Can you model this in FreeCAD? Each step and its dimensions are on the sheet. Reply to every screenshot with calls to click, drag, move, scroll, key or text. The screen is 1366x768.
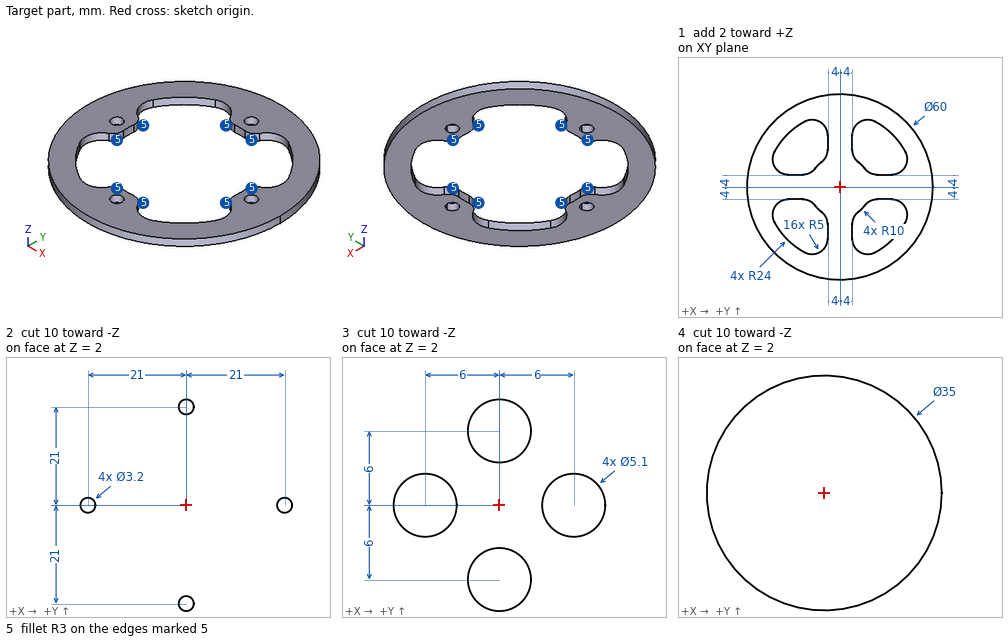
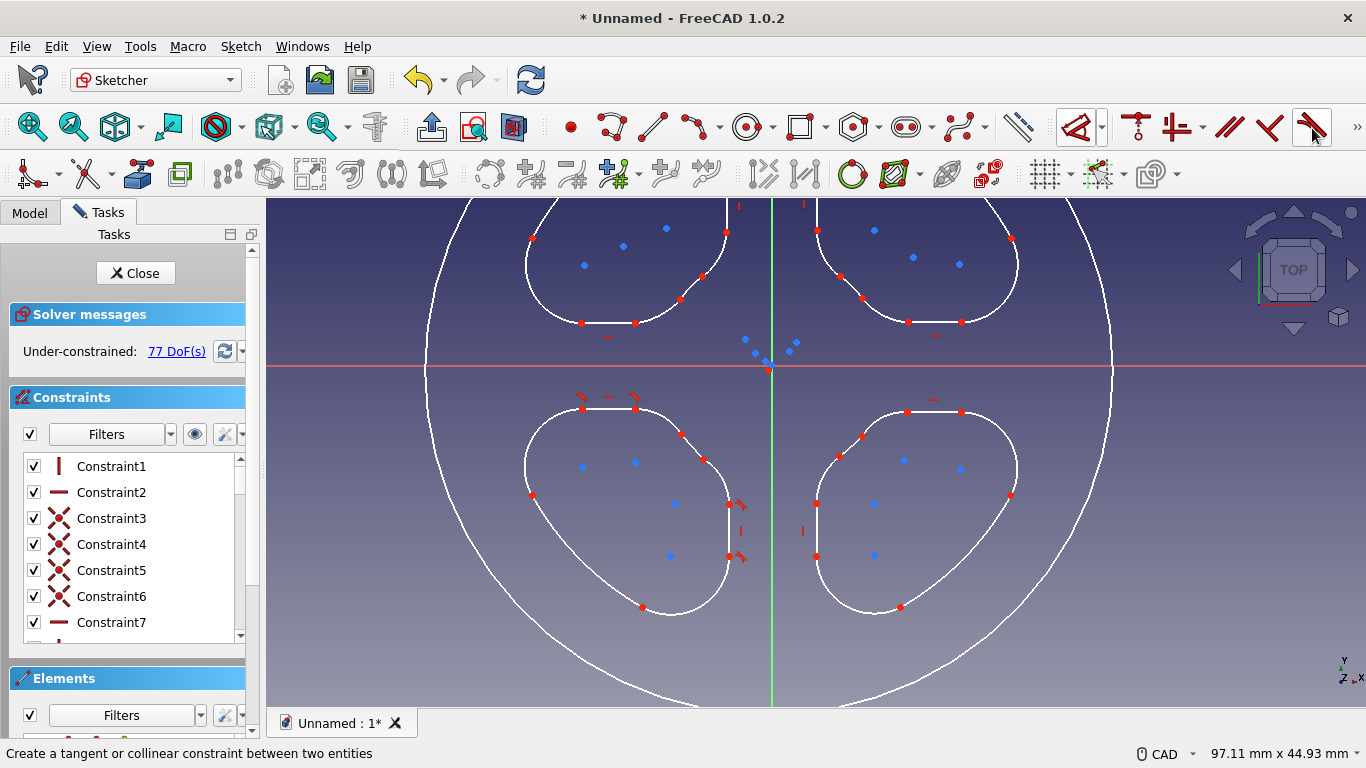
click(678, 614)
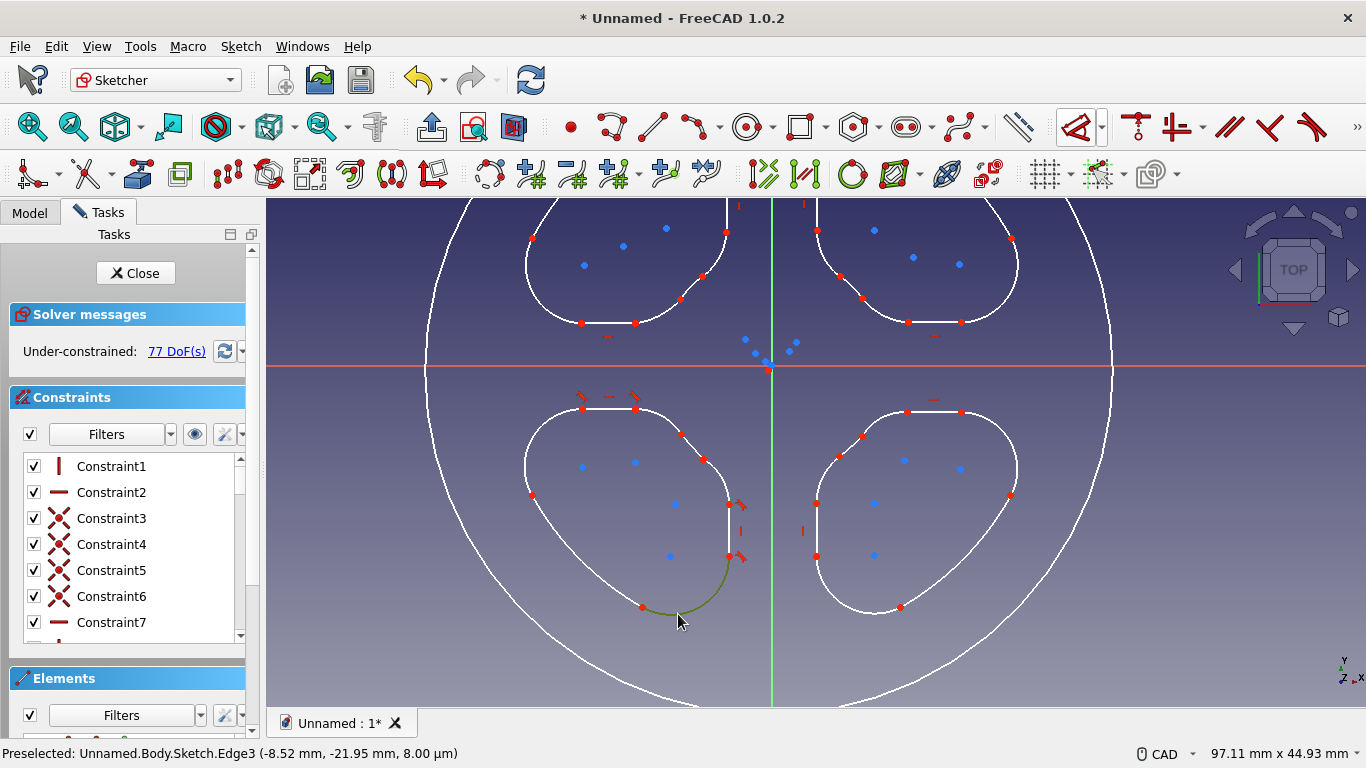
click(559, 535)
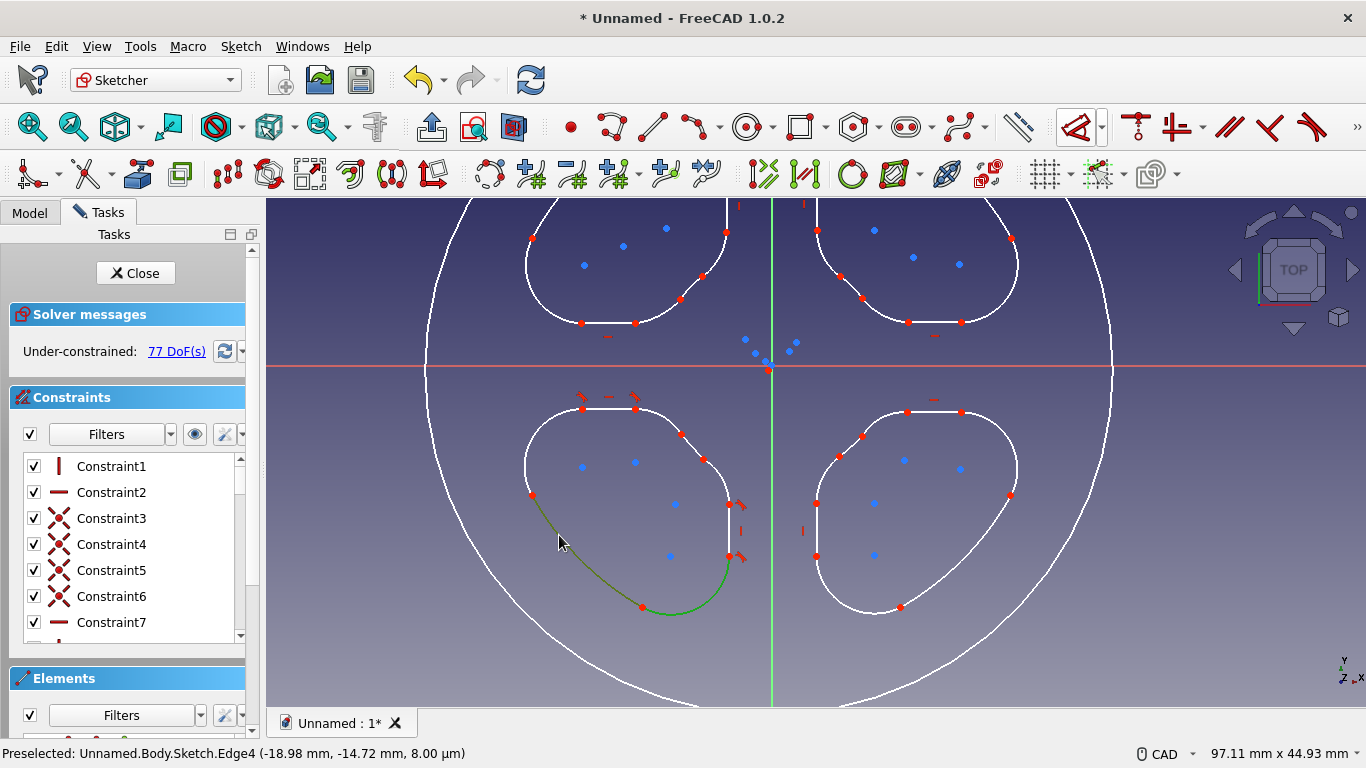
click(1312, 128)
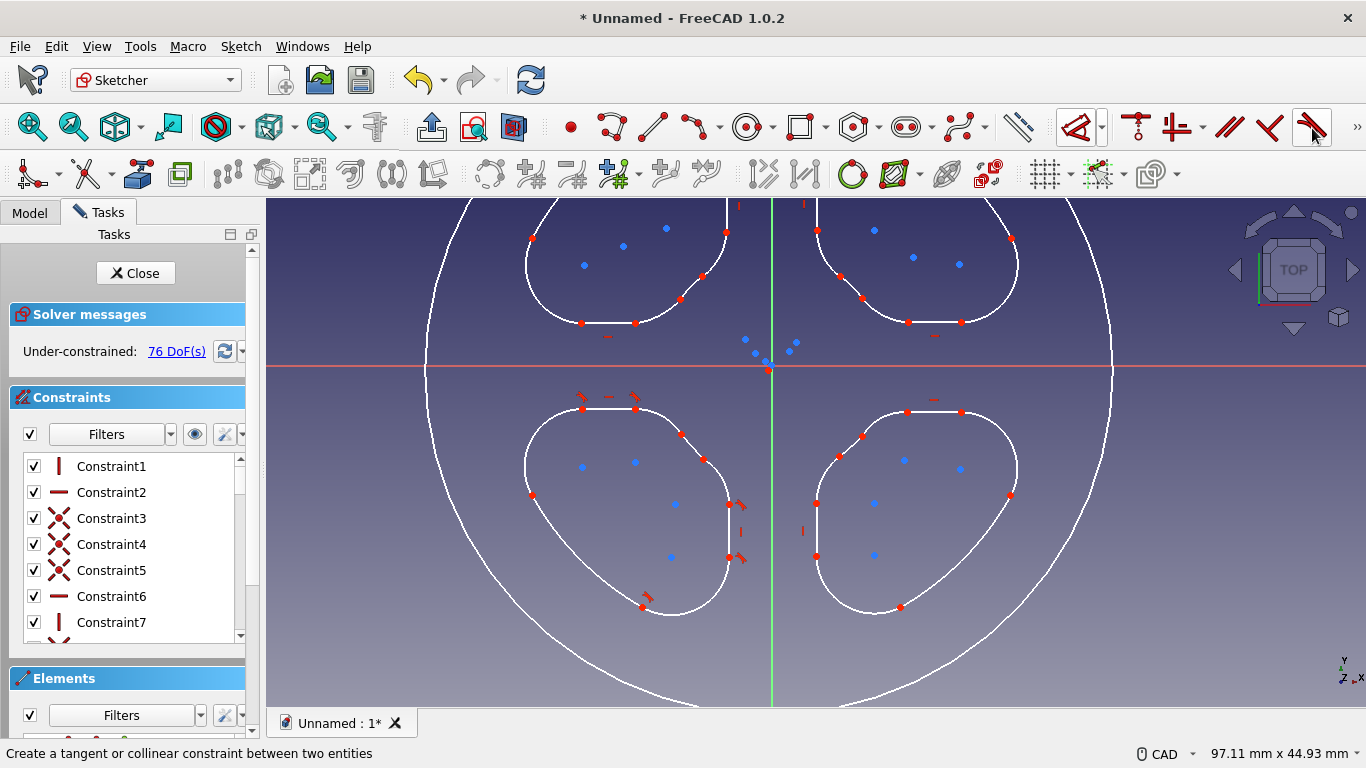
click(559, 535)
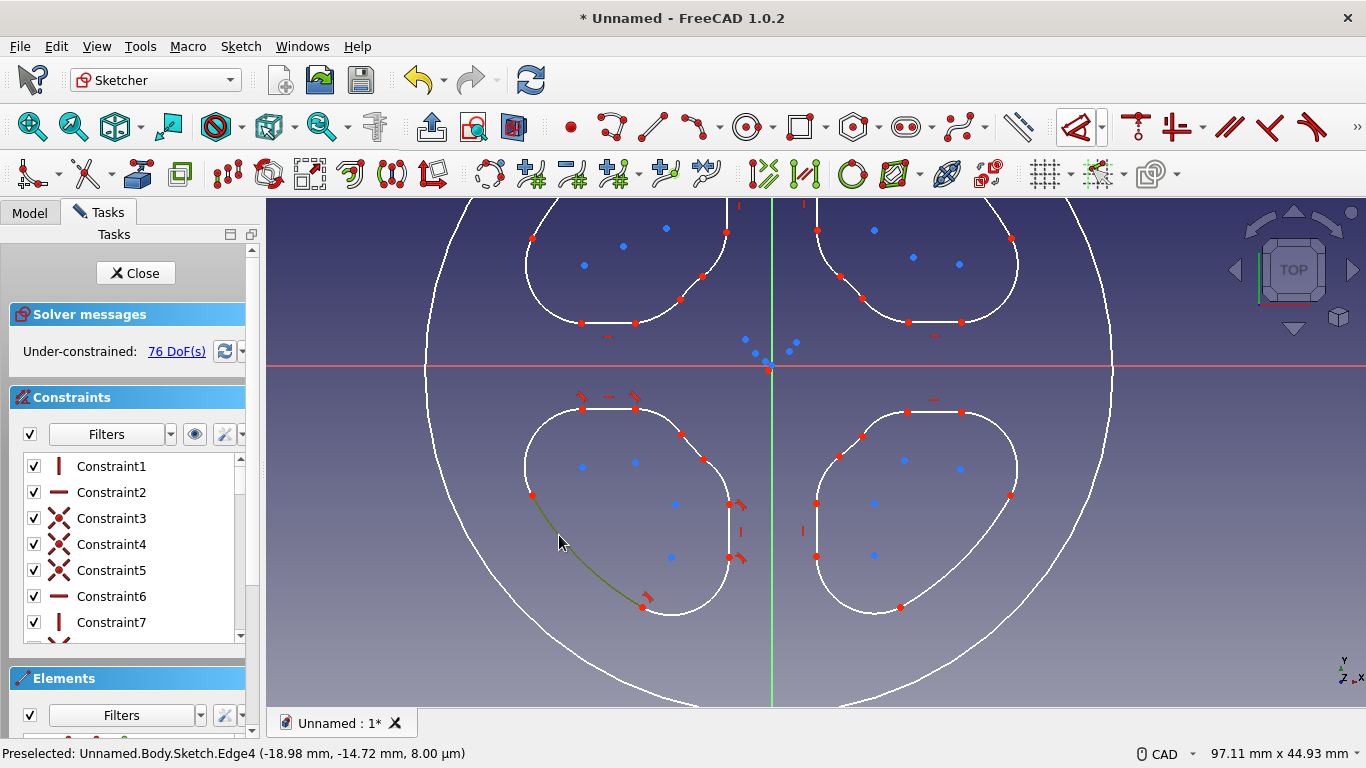
click(549, 420)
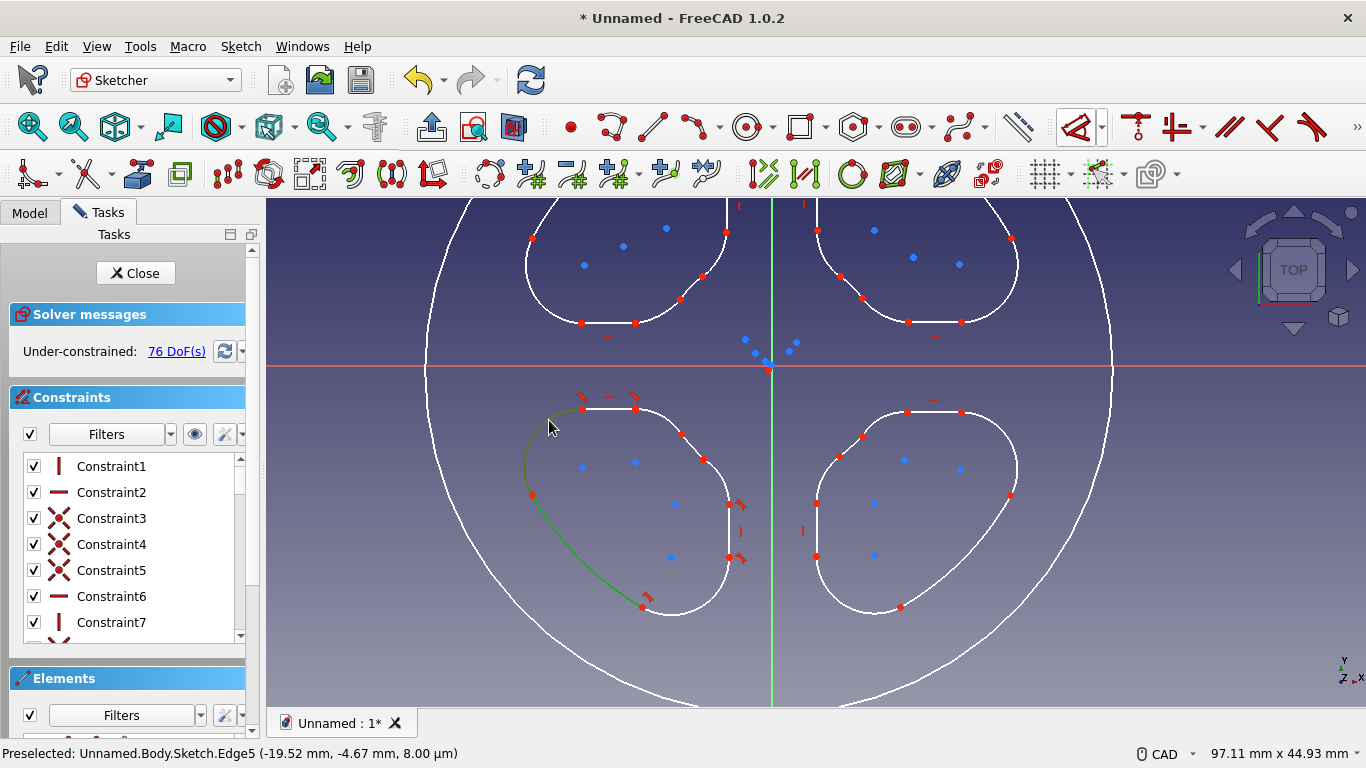
click(1312, 128)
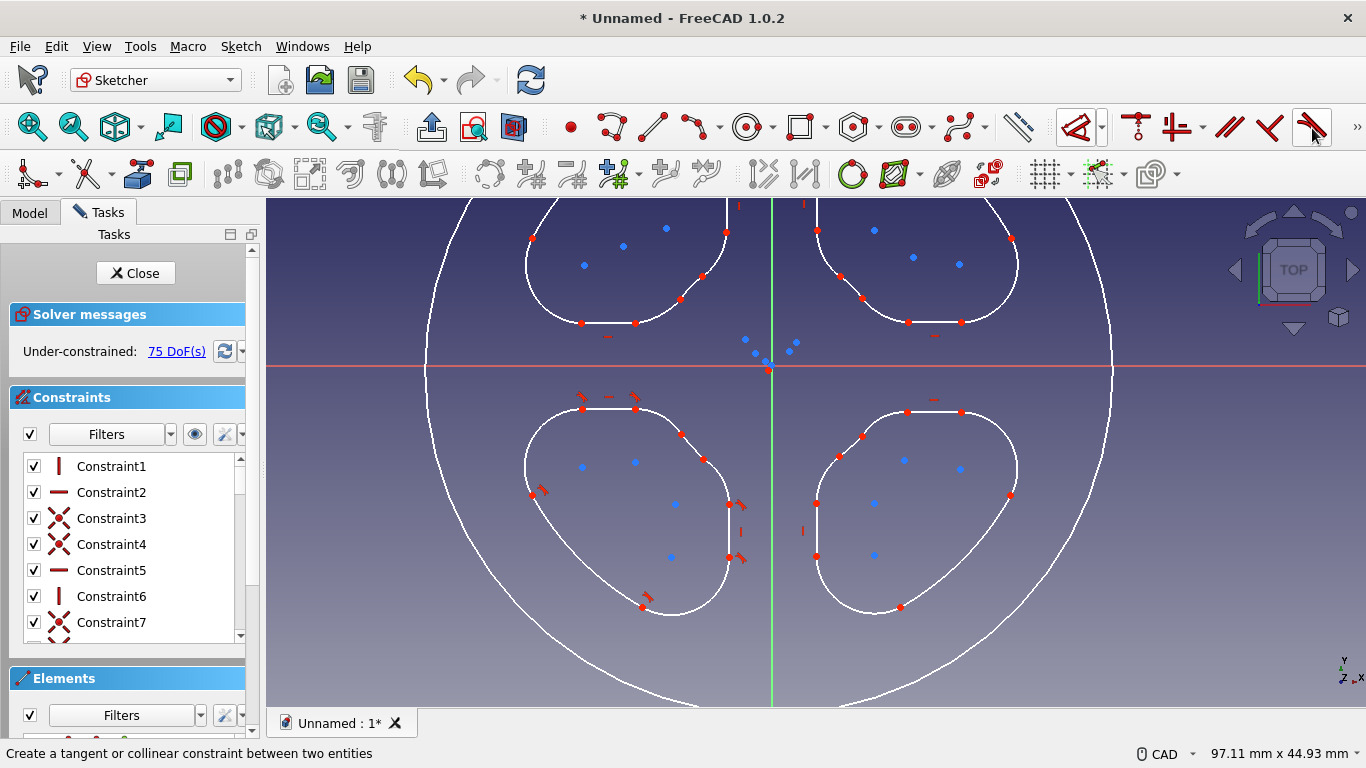
click(671, 422)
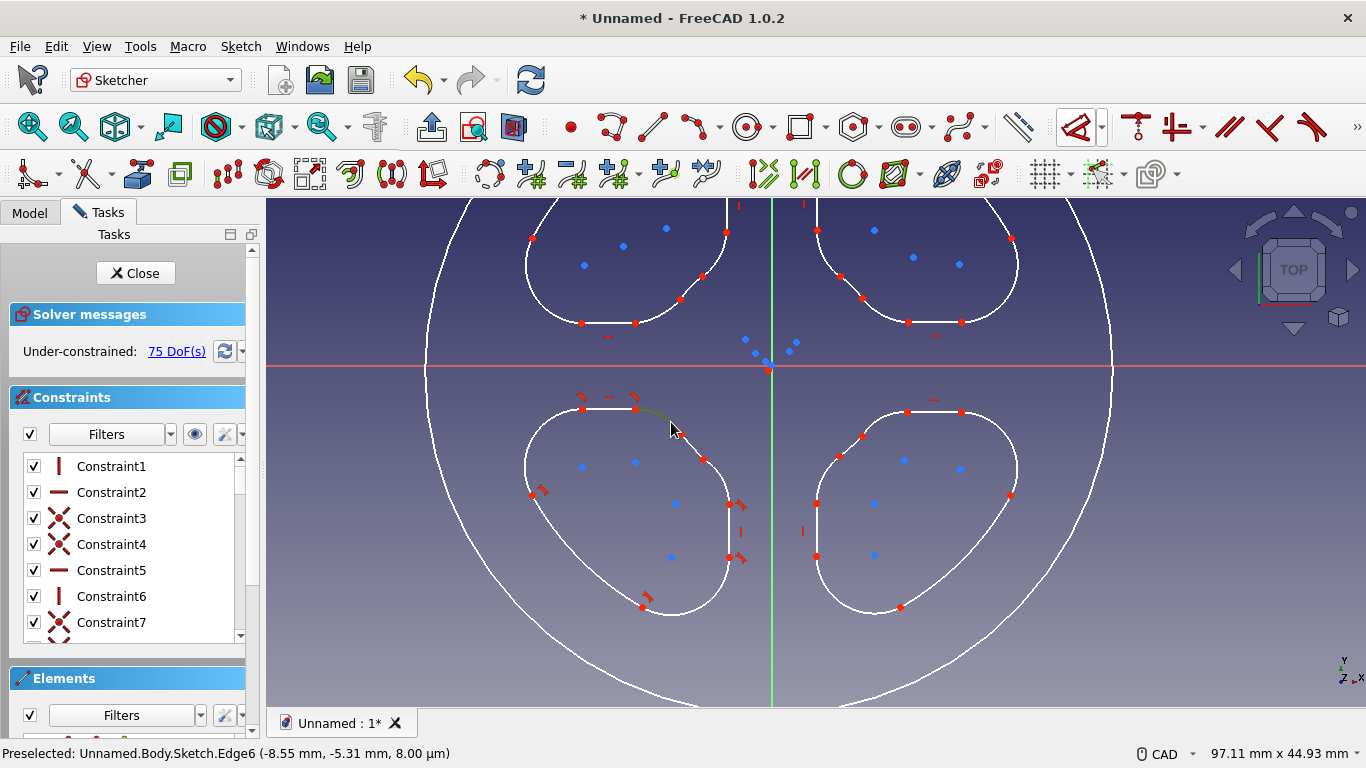
scroll(688, 442, up, 2)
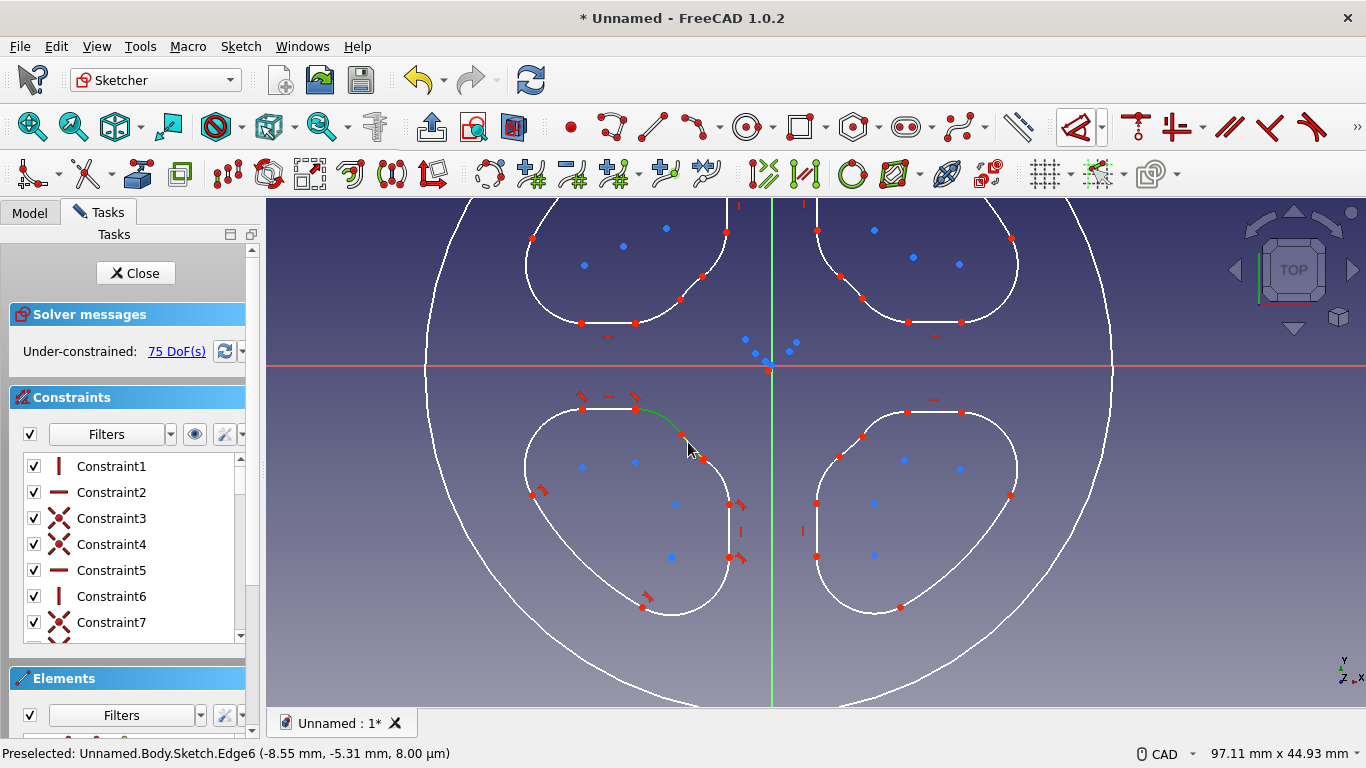
click(688, 442)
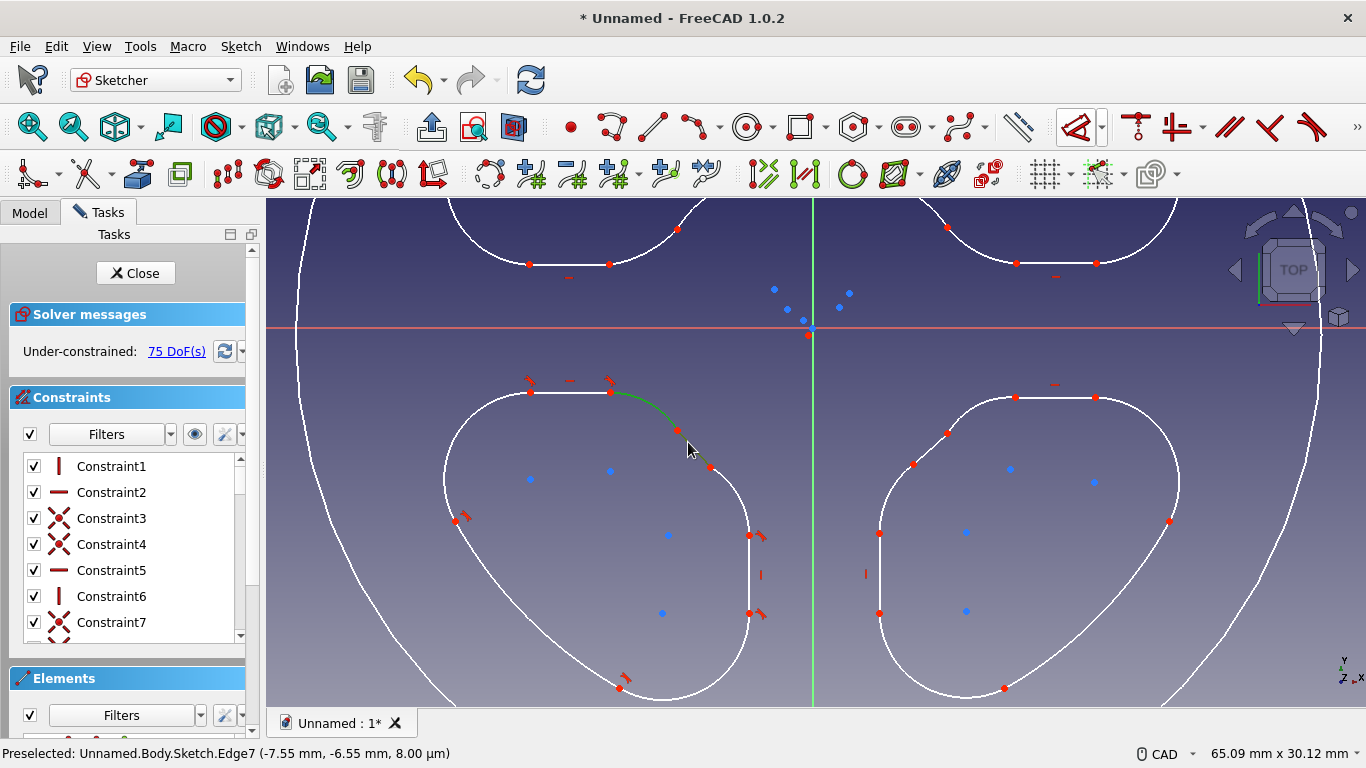
key(t)